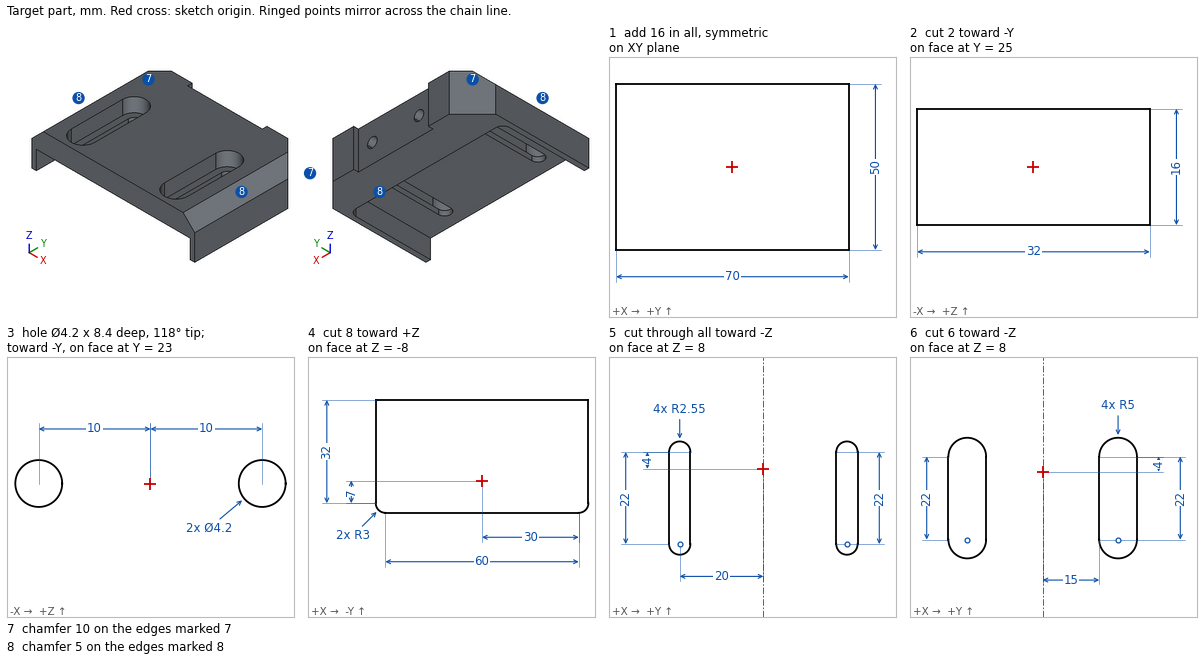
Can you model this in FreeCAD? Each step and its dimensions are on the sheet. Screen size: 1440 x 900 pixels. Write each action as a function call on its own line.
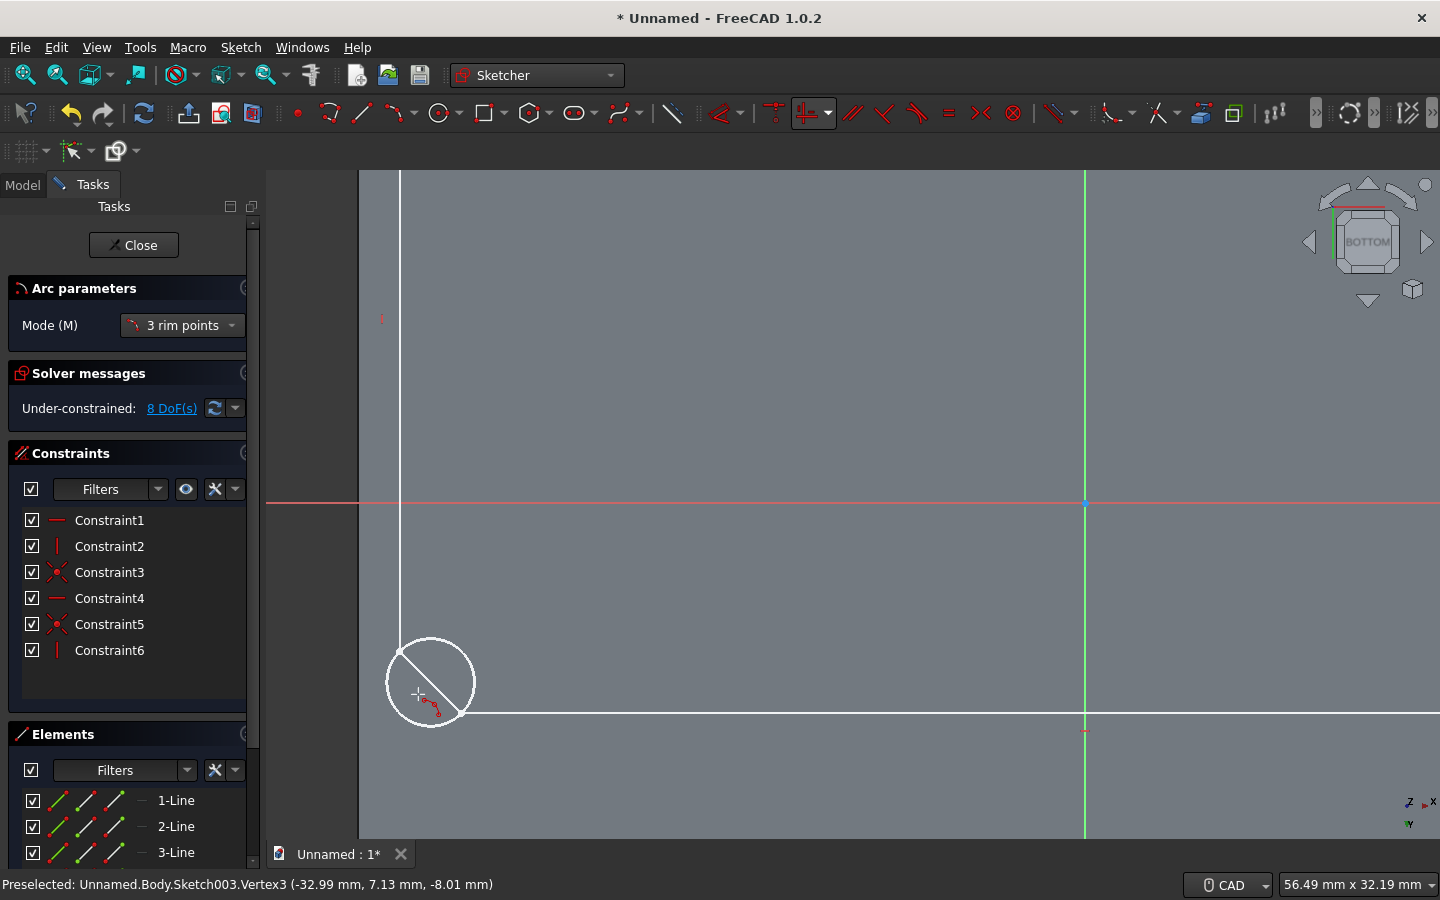
click(418, 693)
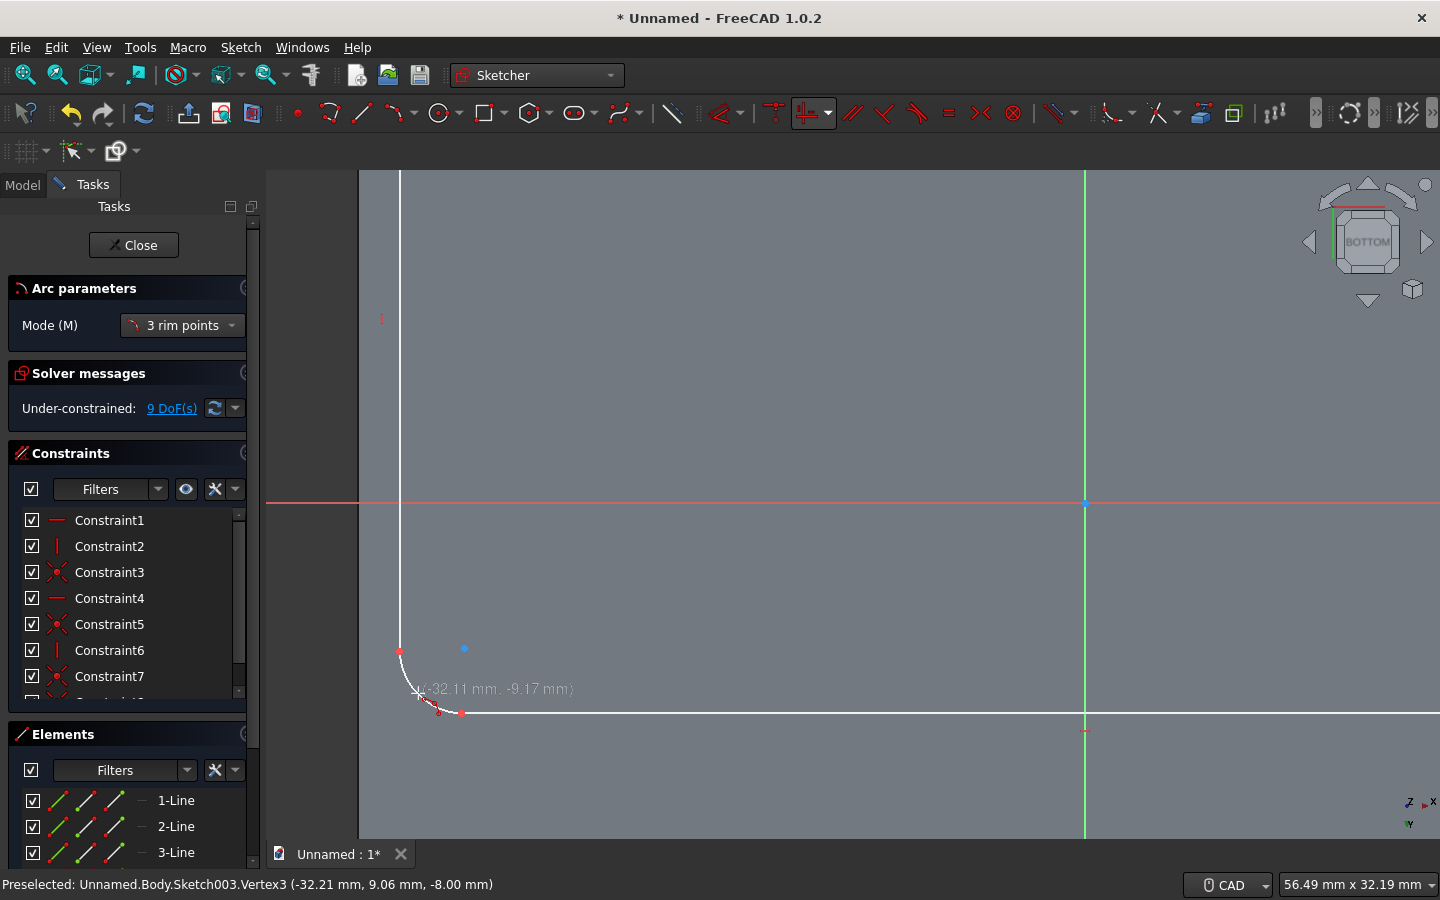
scroll(419, 696, down, 3)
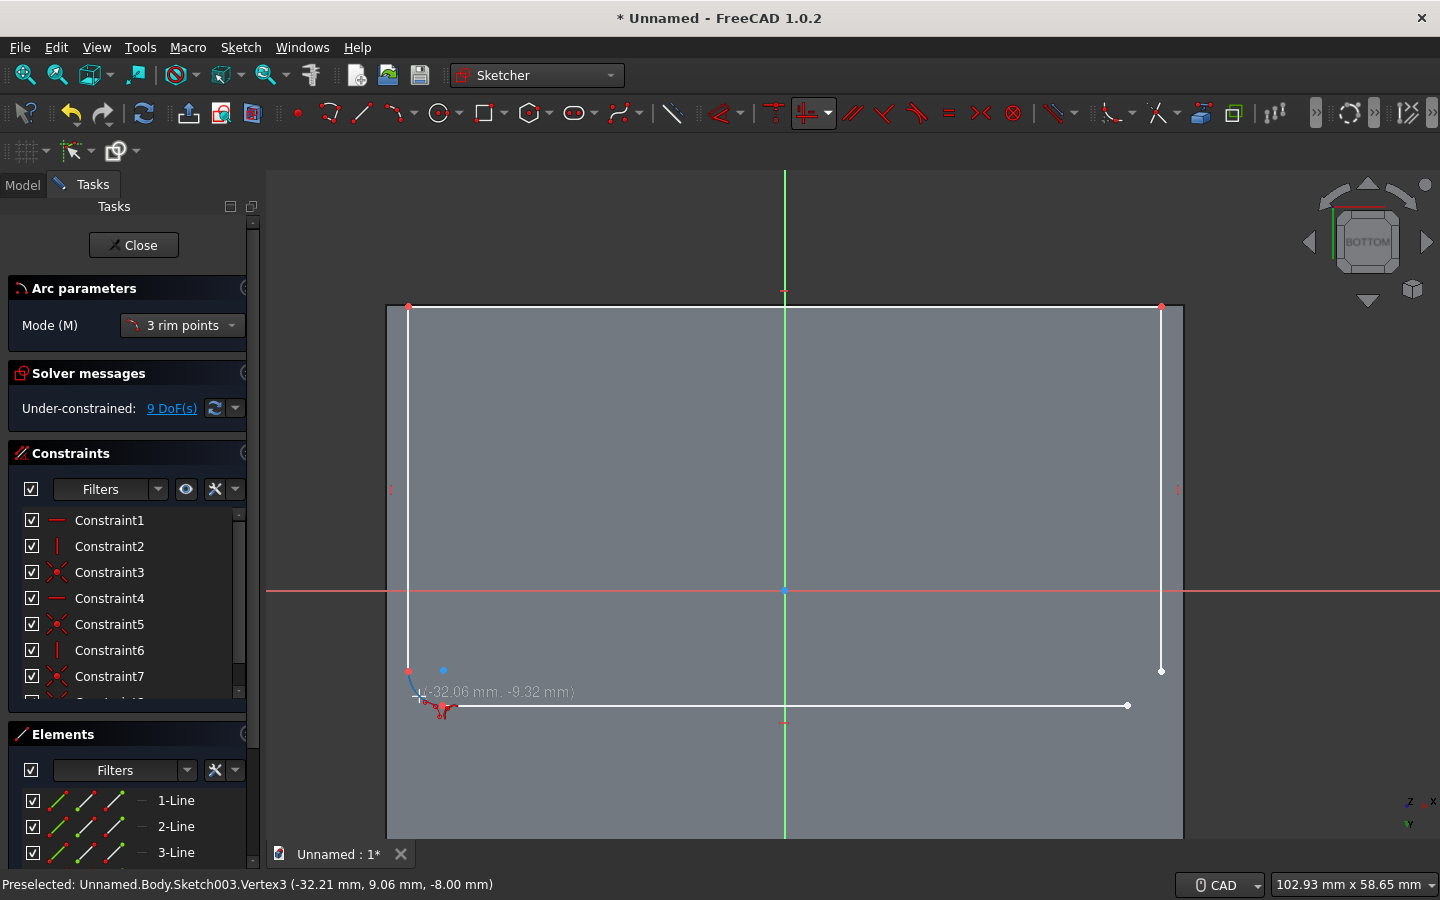
click(1161, 672)
click(1127, 706)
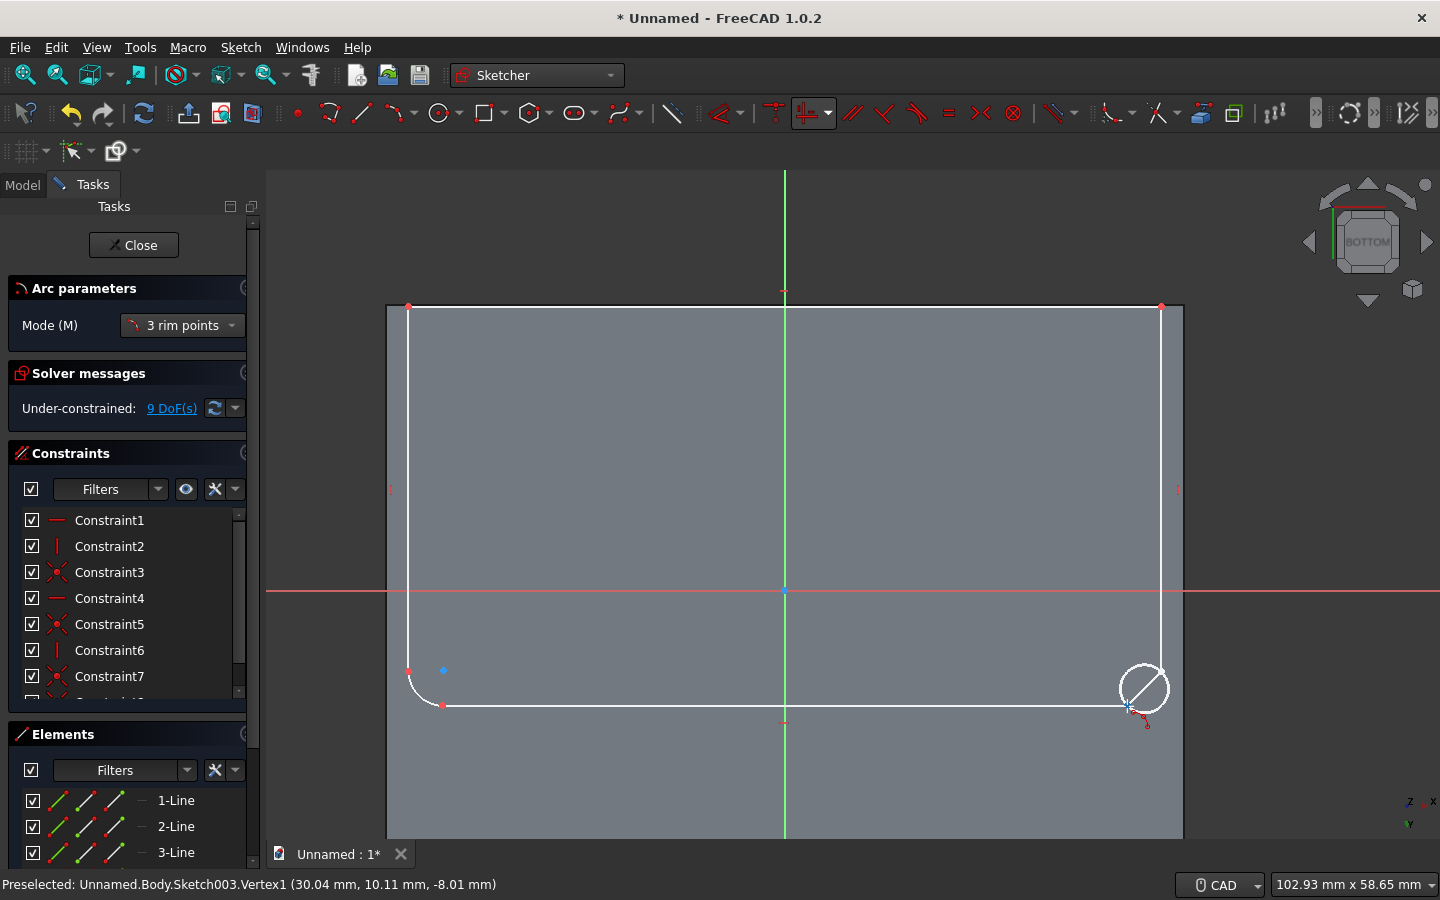
scroll(1151, 695, up, 3)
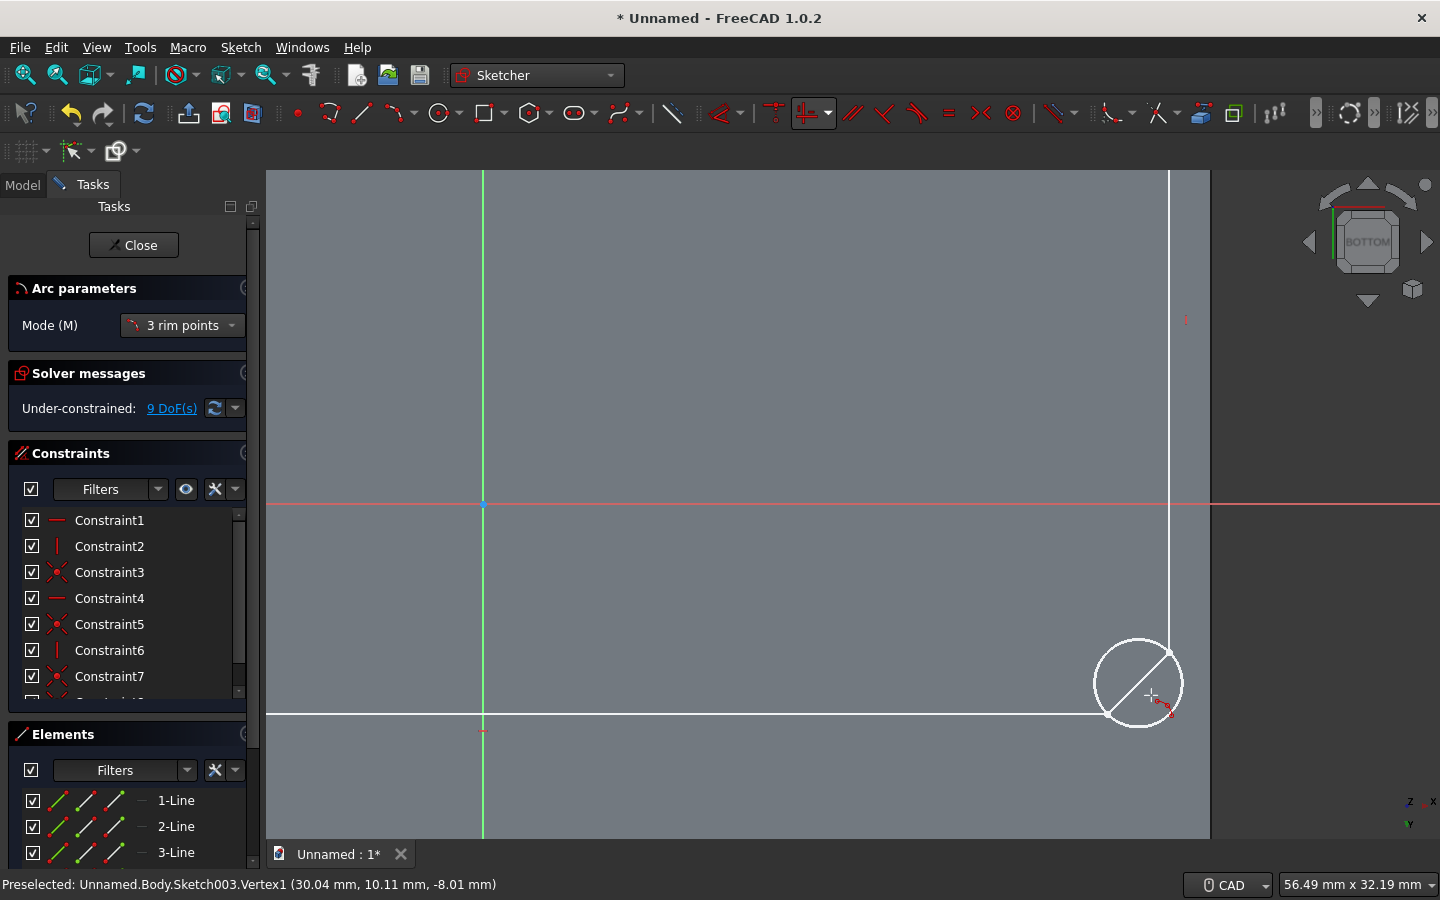
click(1151, 694)
key(Escape)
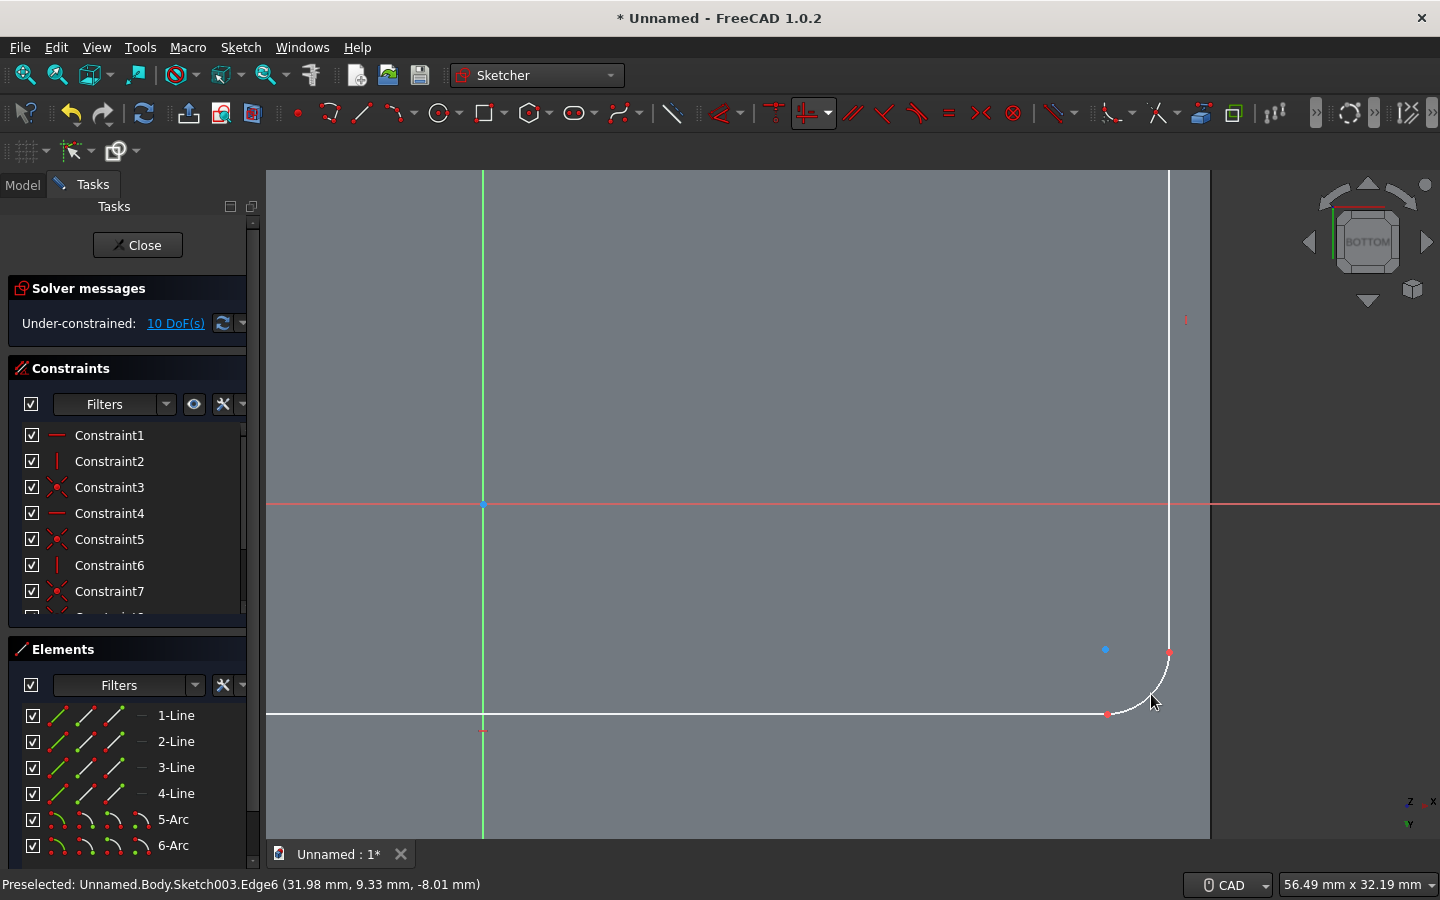
click(733, 714)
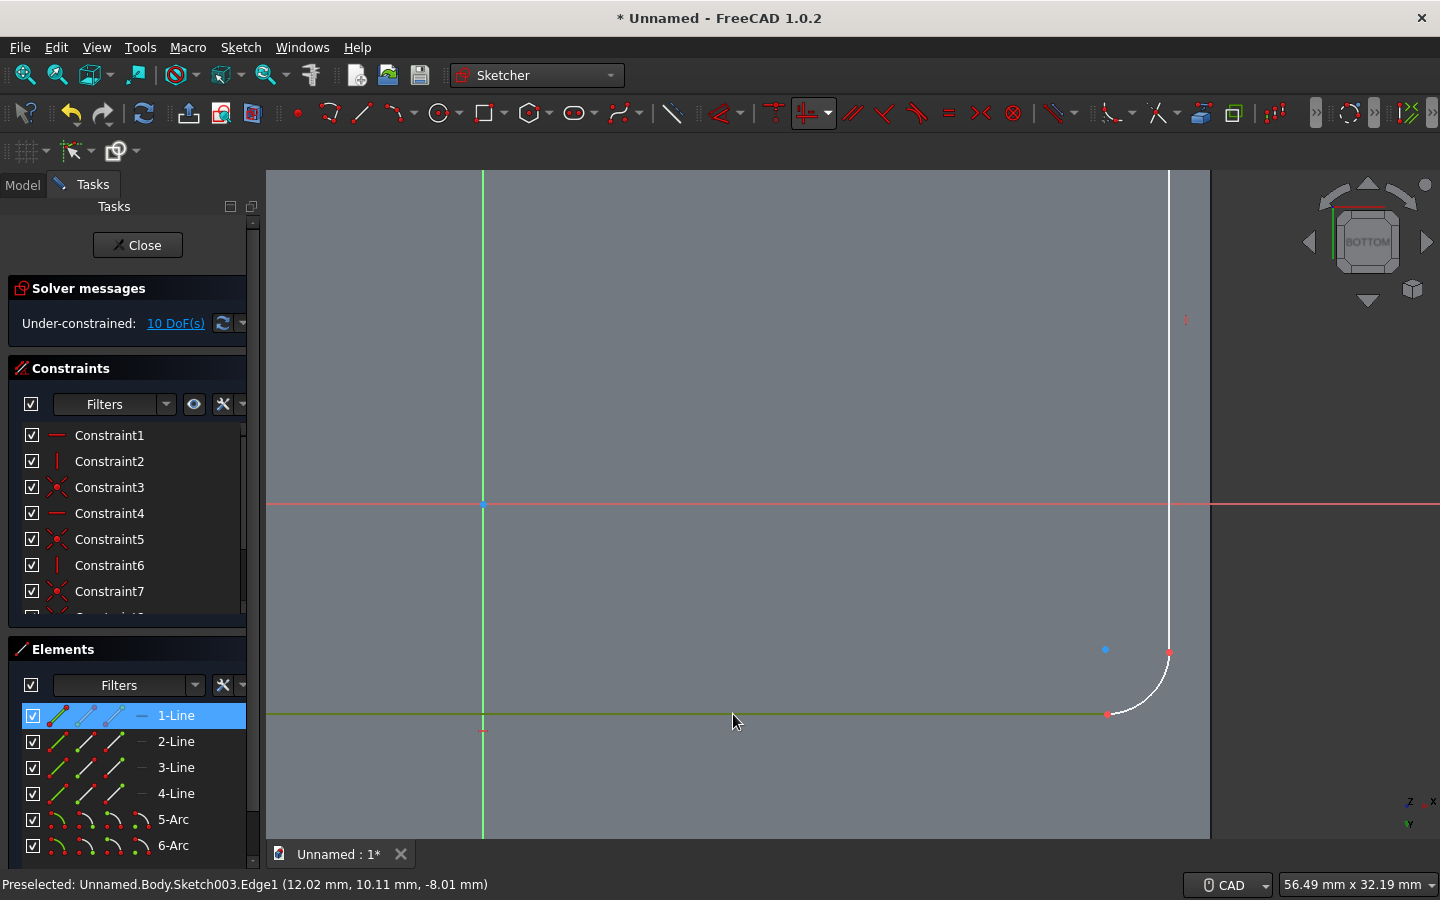
scroll(1151, 695, down, 3)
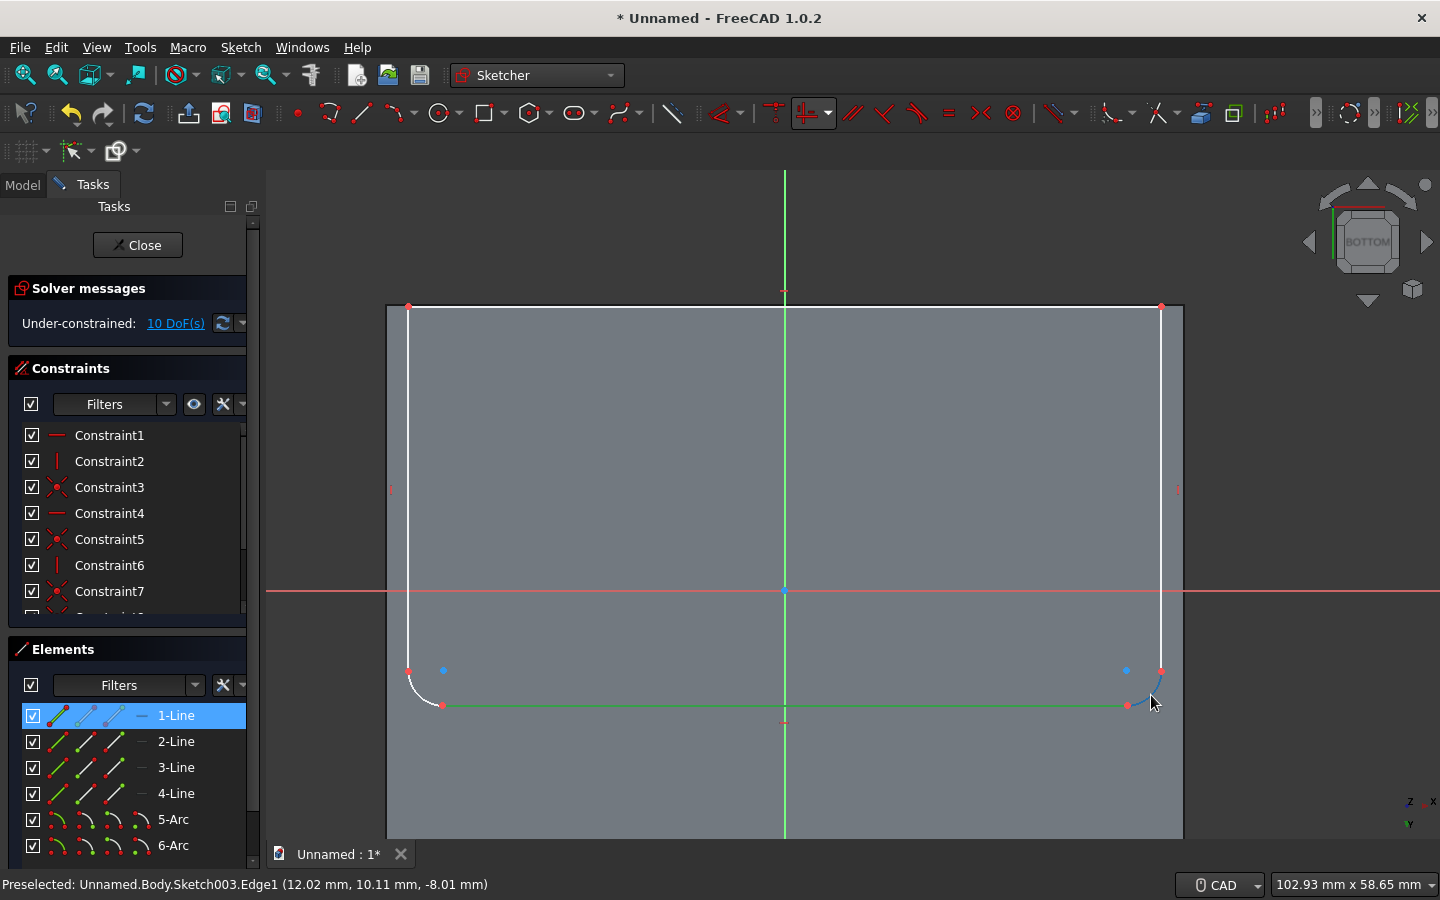
click(413, 687)